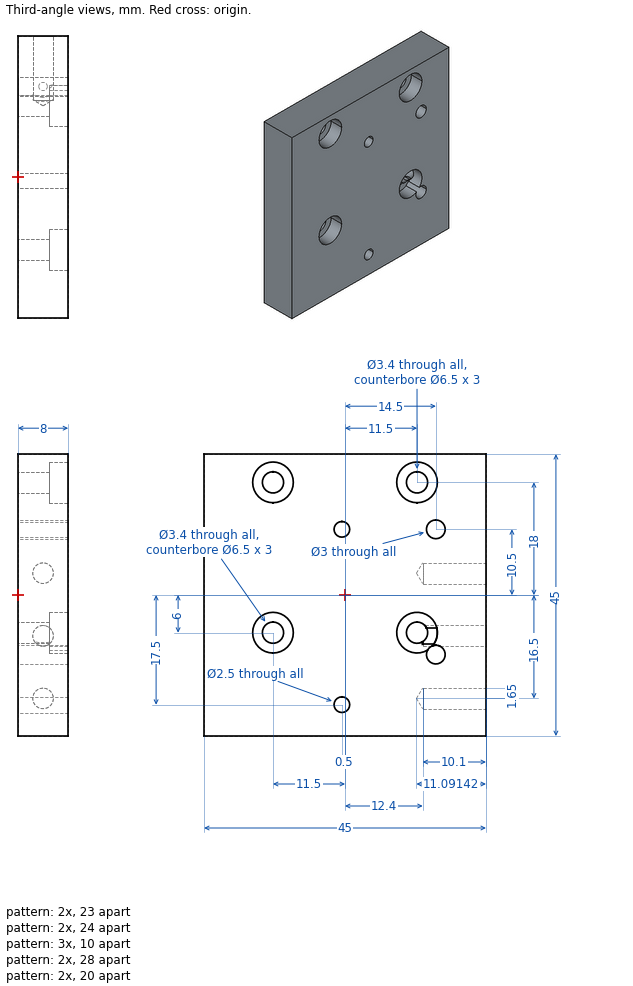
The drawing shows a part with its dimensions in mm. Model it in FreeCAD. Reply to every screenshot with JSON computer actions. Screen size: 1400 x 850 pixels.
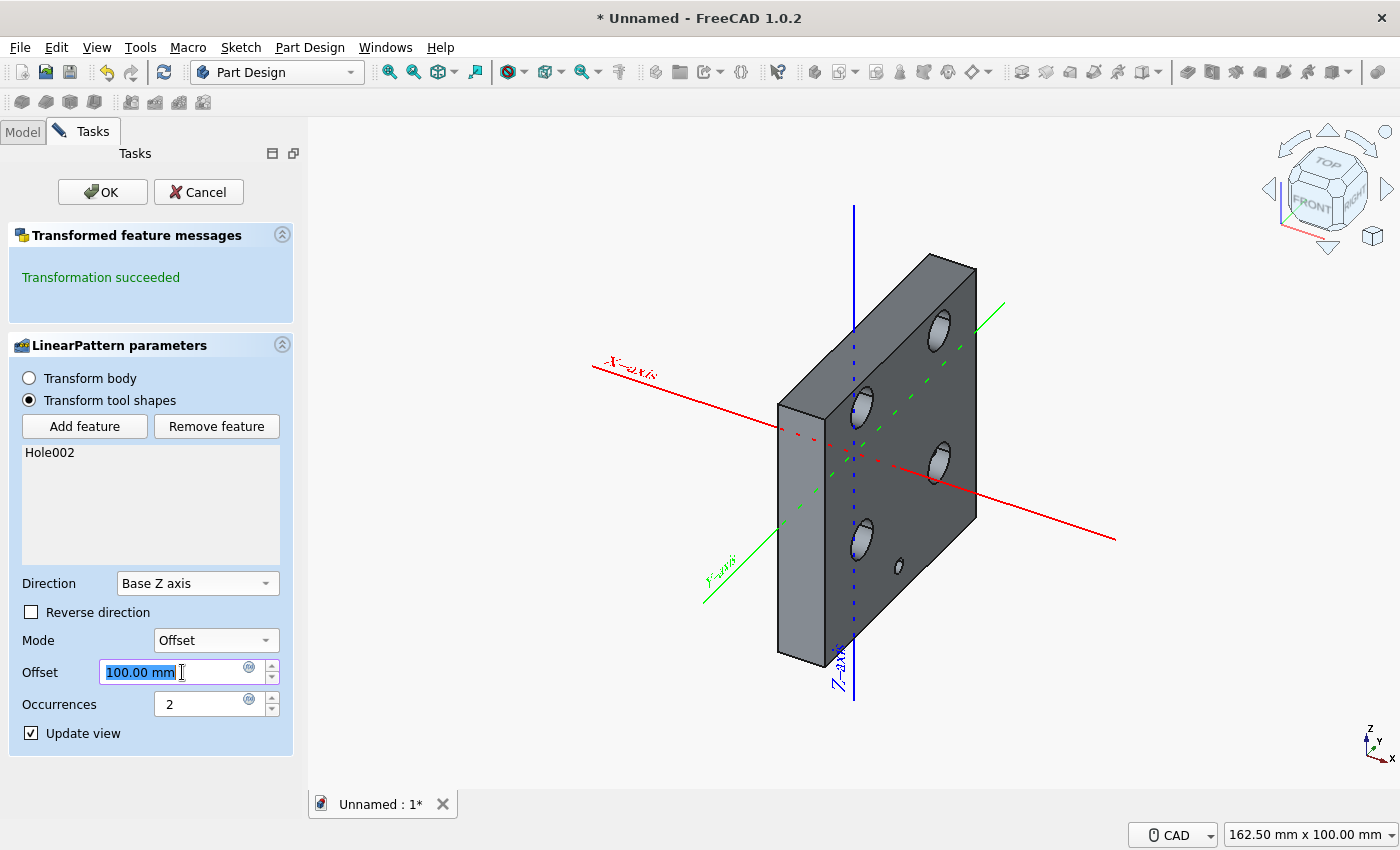
{"action": "type", "text": "28"}
{"action": "key", "text": "Tab"}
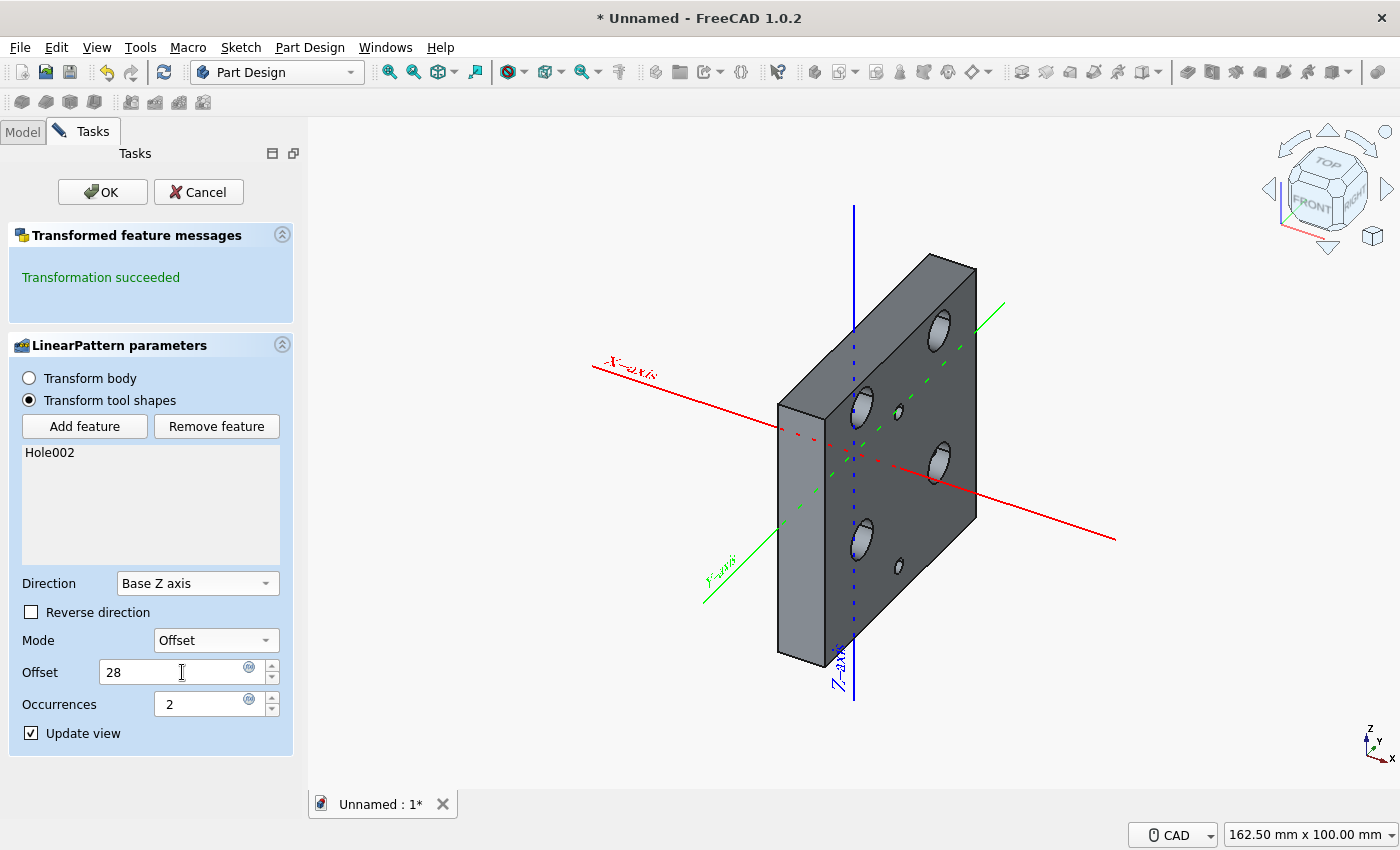
{"action": "triple_click", "coordinate": [209, 704]}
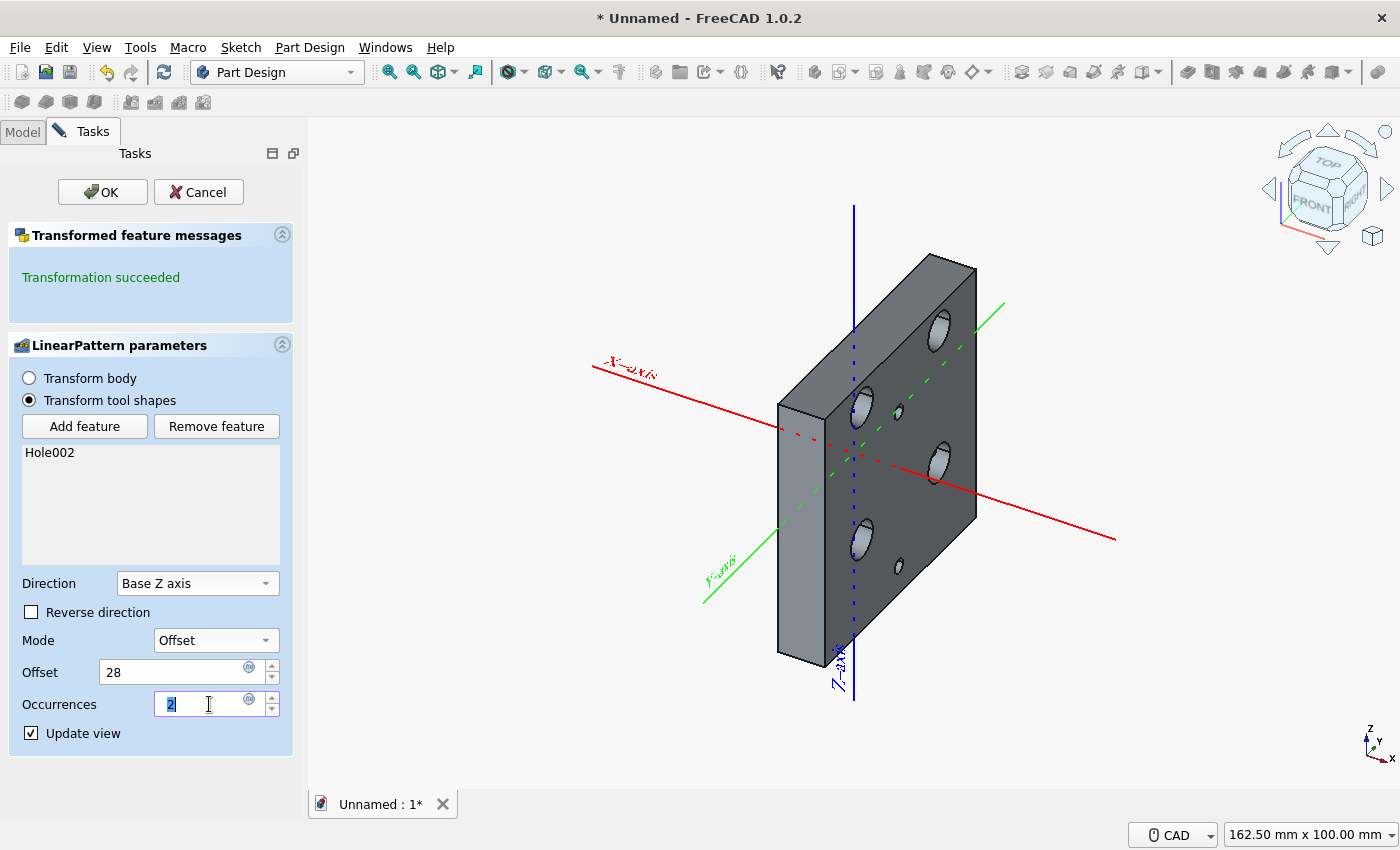
{"action": "type", "text": "2"}
{"action": "key", "text": "Tab"}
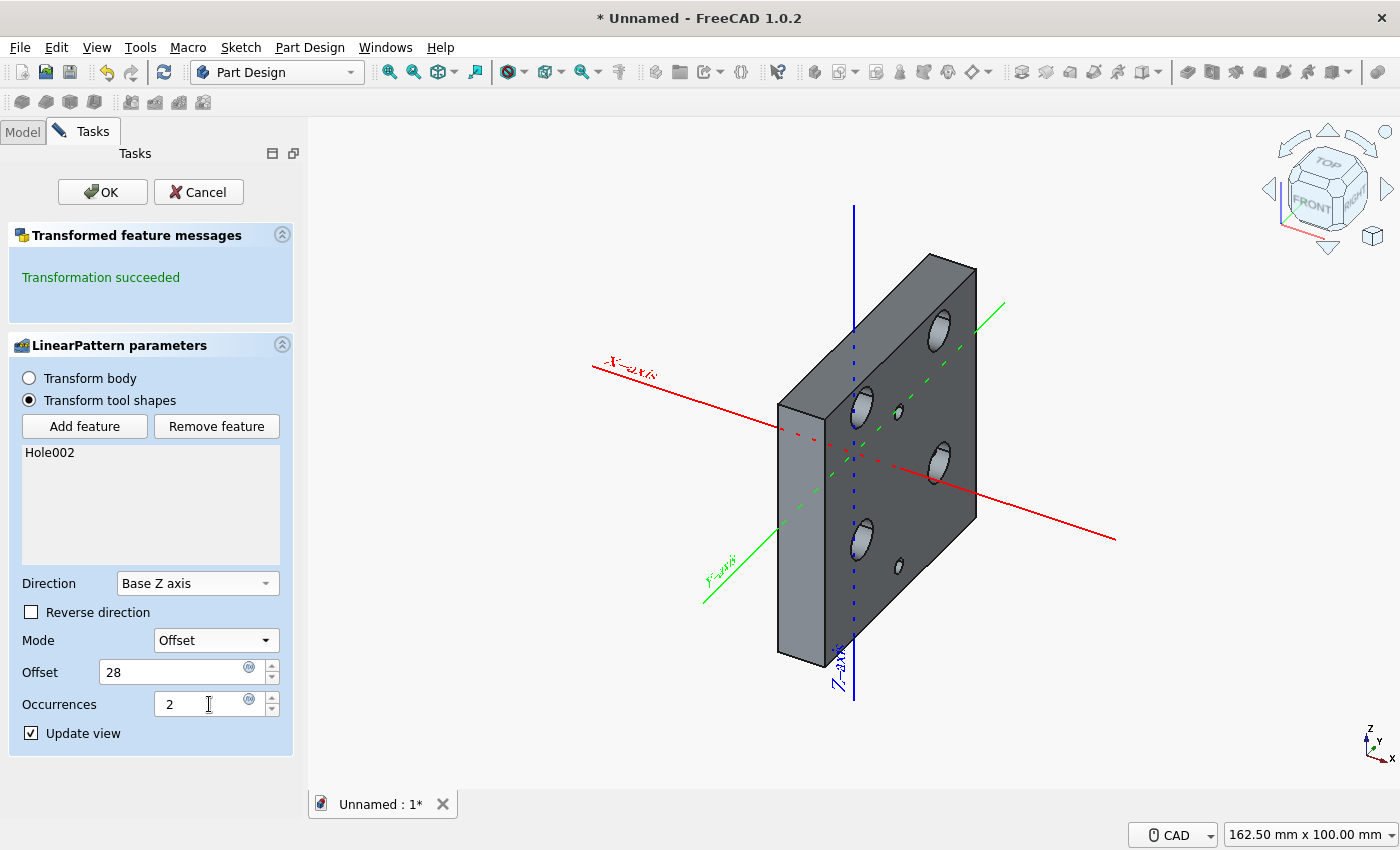
{"action": "left_click", "coordinate": [103, 192]}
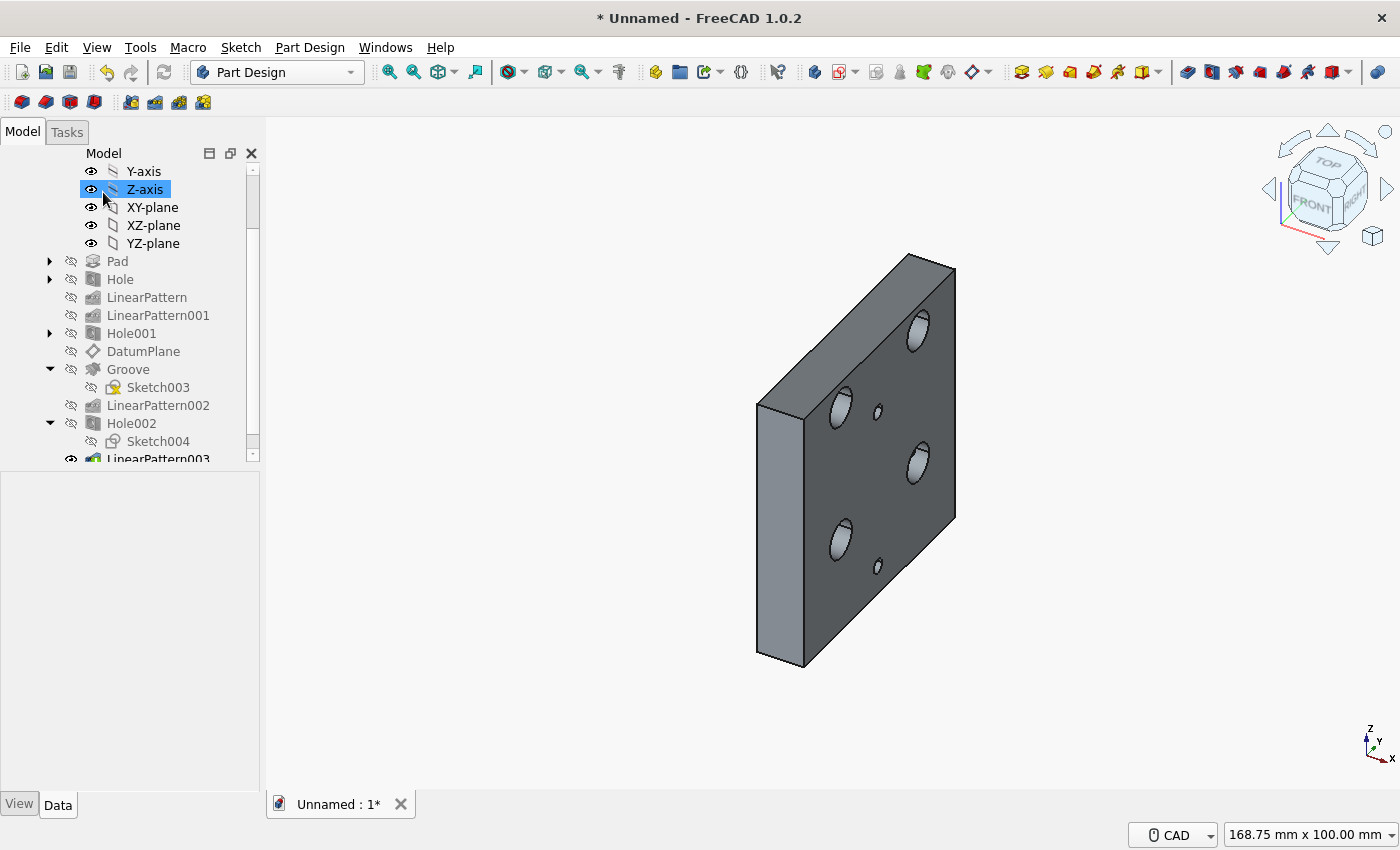
{"action": "left_click", "coordinate": [880, 467]}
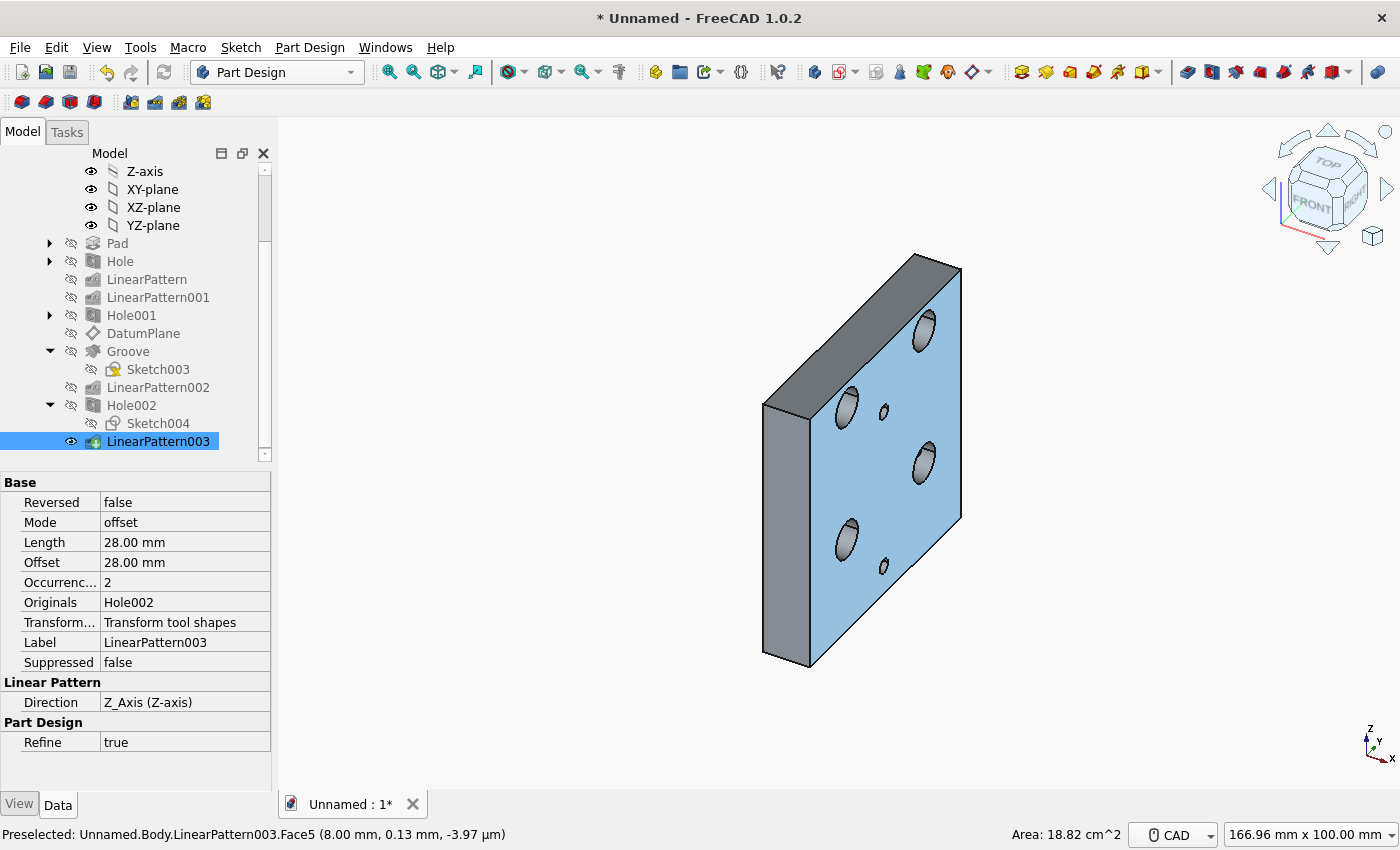
{"action": "left_click", "coordinate": [840, 72]}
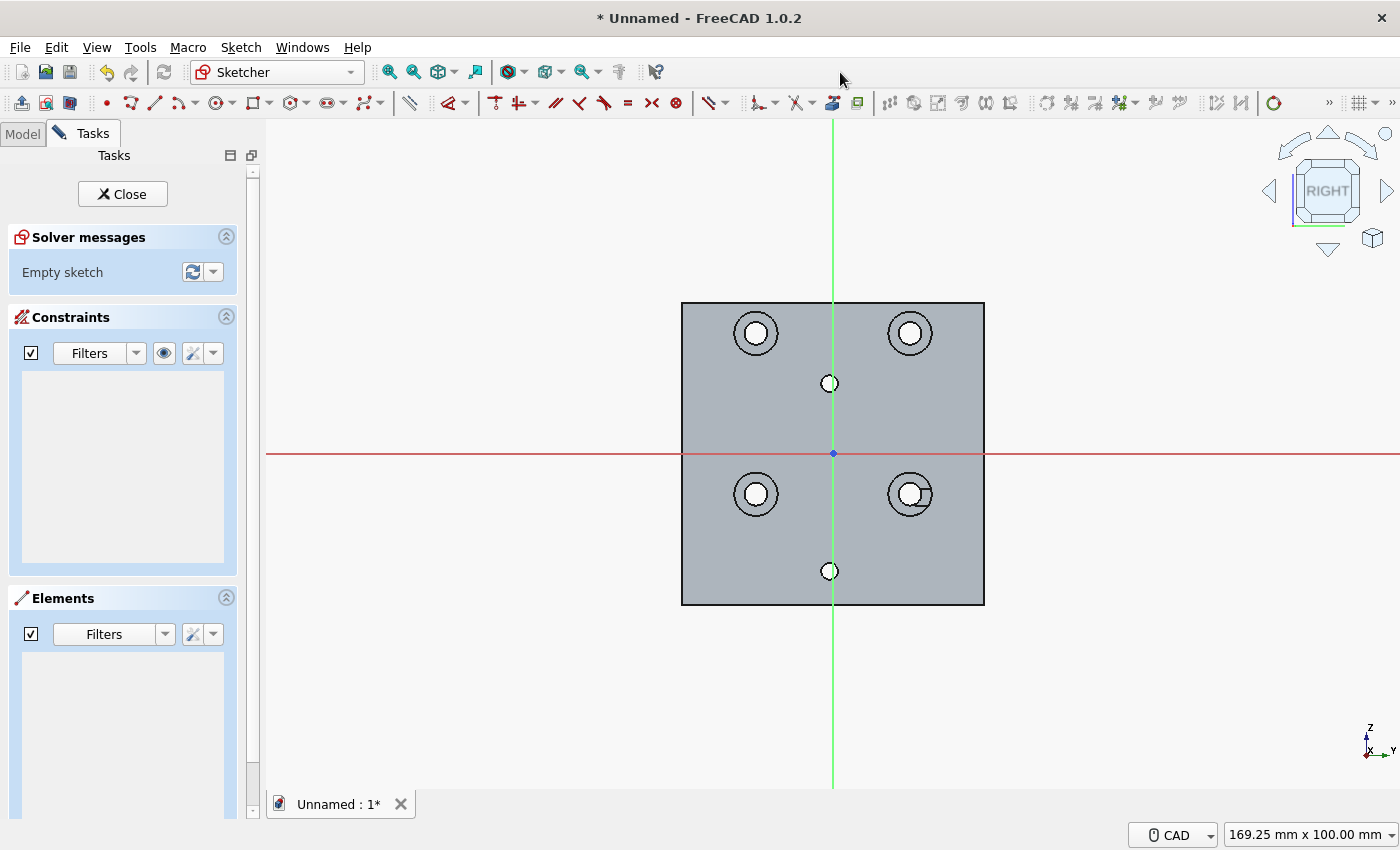
{"action": "scroll", "coordinate": [939, 380], "scroll_direction": "up", "scroll_amount": 15}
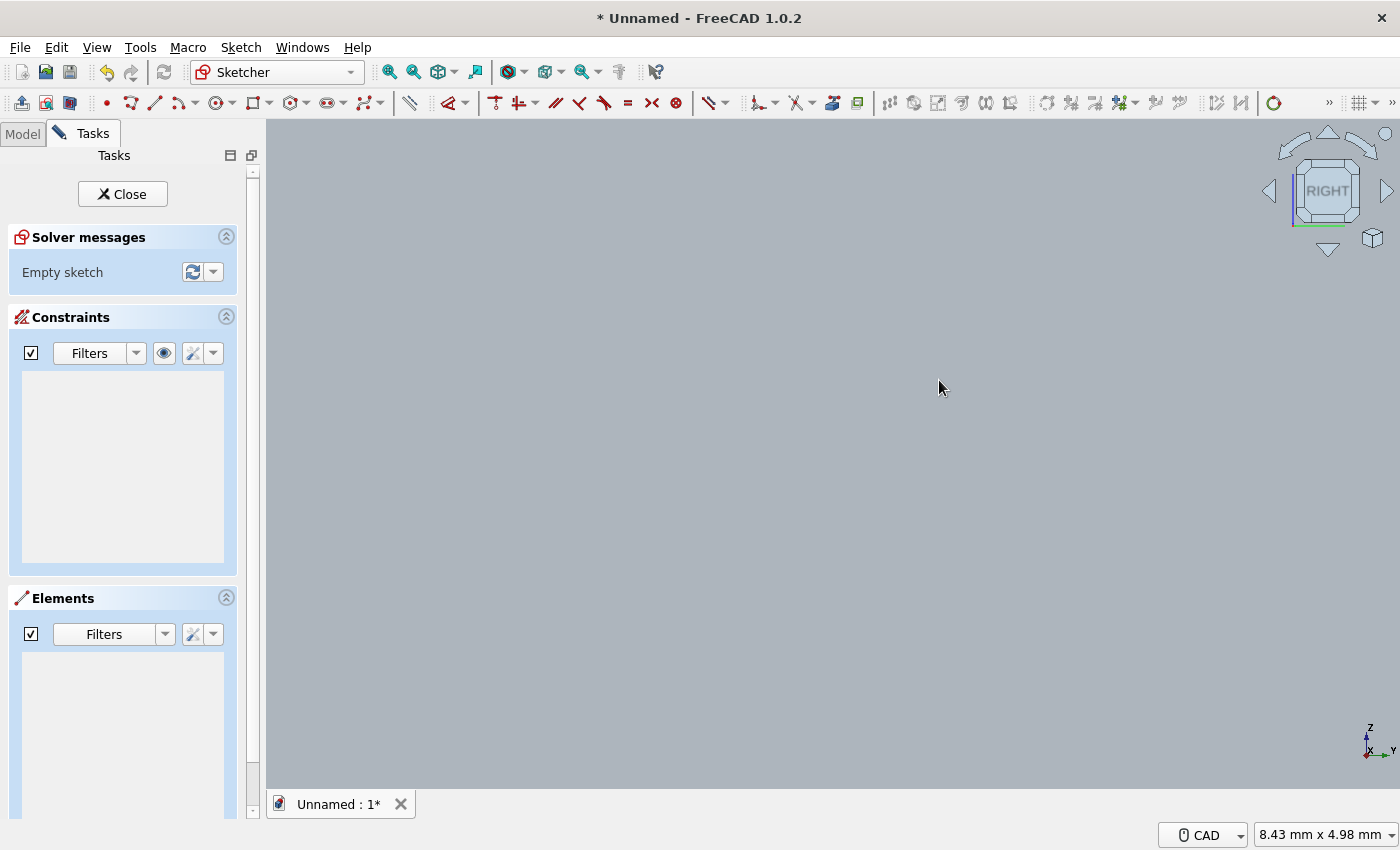
{"action": "key", "text": "g c"}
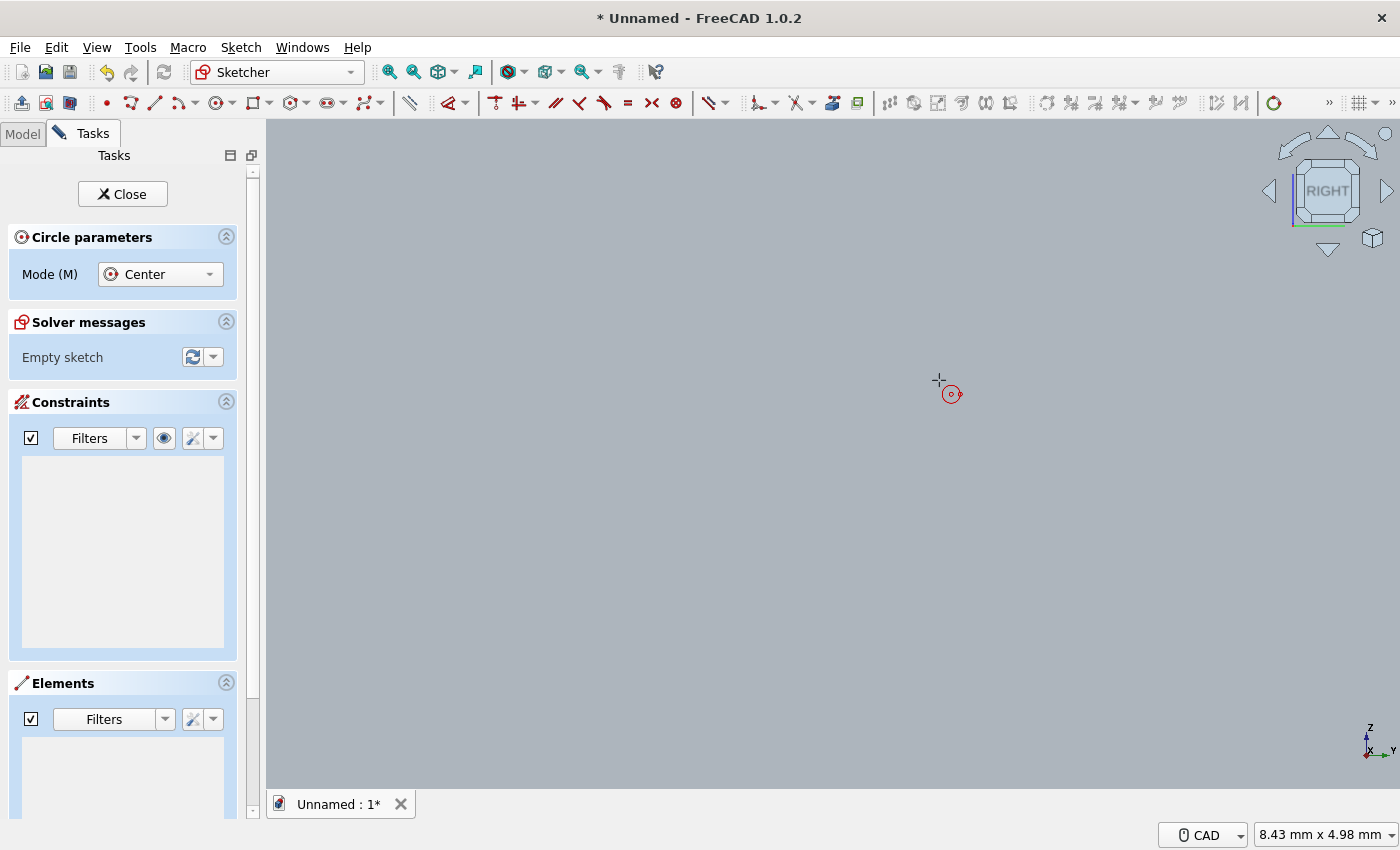
{"action": "left_click", "coordinate": [750, 446]}
{"action": "left_click", "coordinate": [893, 303]}
{"action": "key", "text": "Escape"}